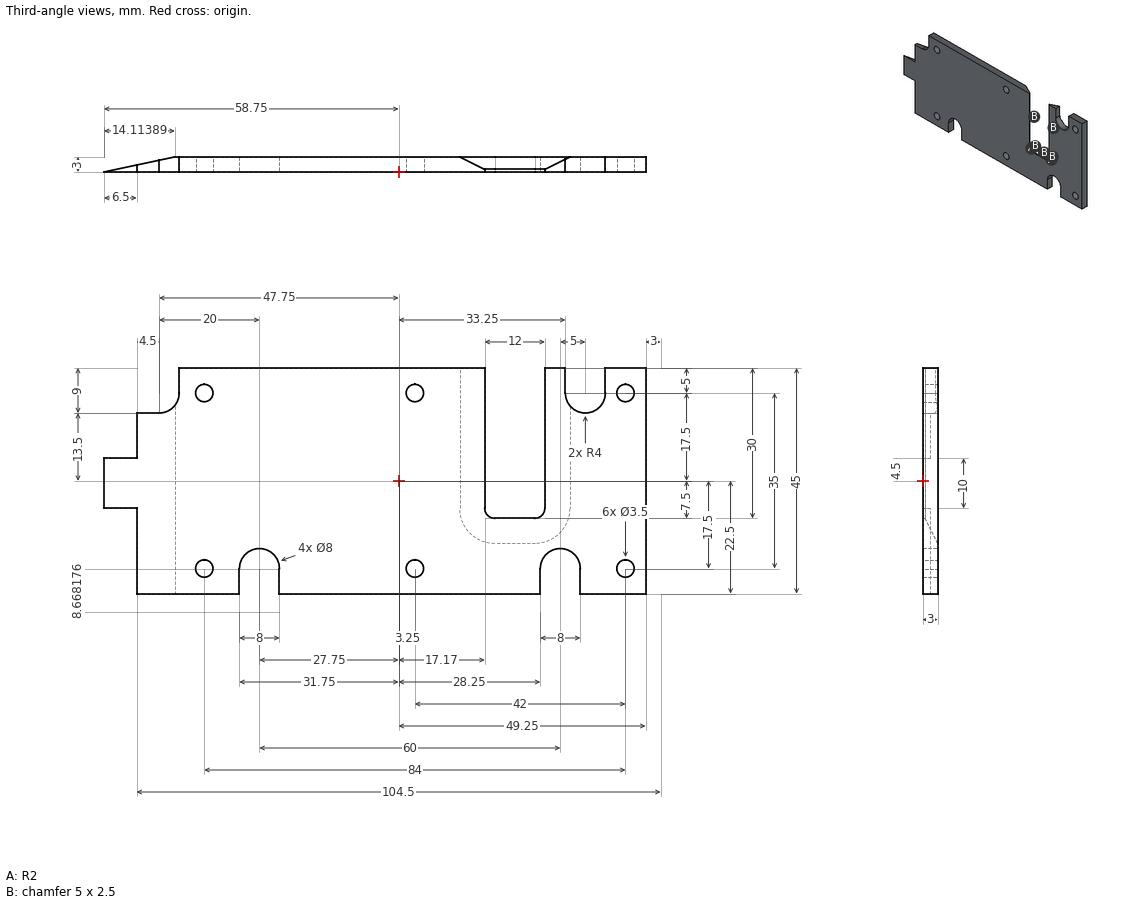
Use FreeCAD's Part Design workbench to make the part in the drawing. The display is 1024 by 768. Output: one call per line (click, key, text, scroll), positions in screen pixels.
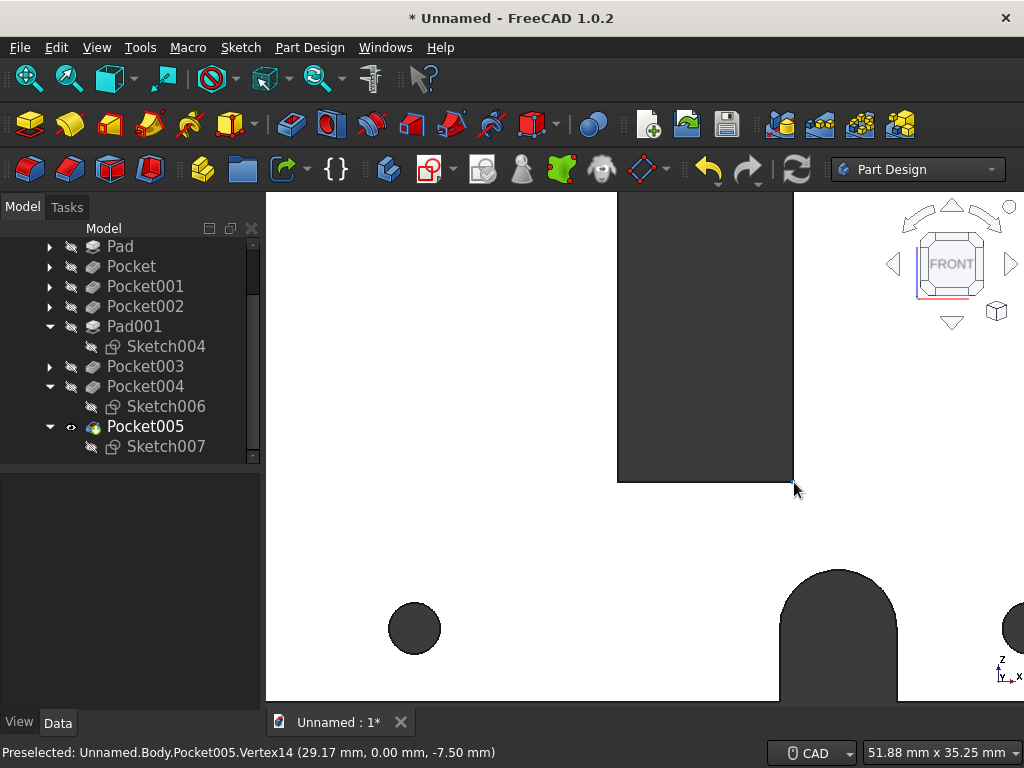
click(30, 80)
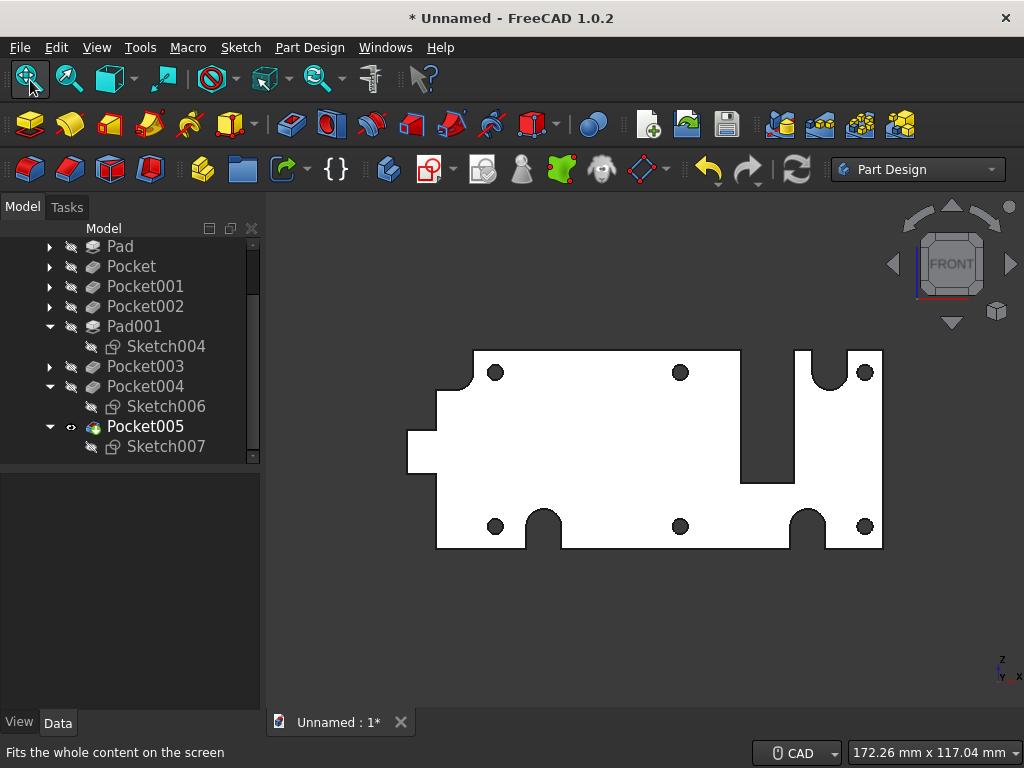
key(3)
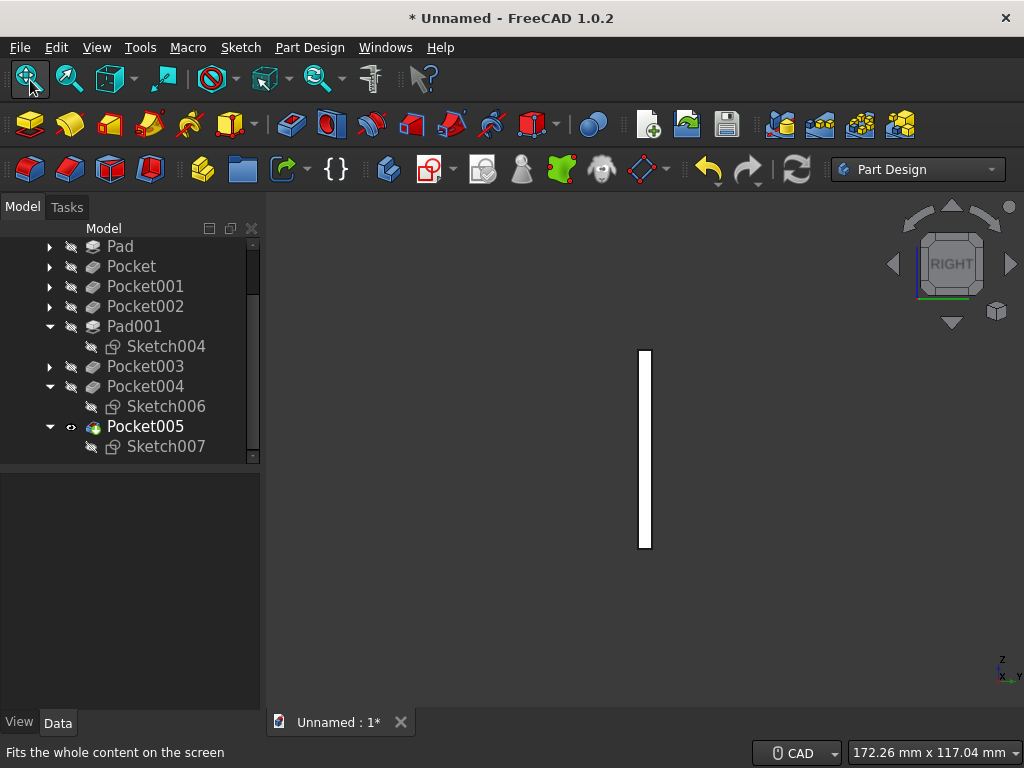
key(v)
key(f)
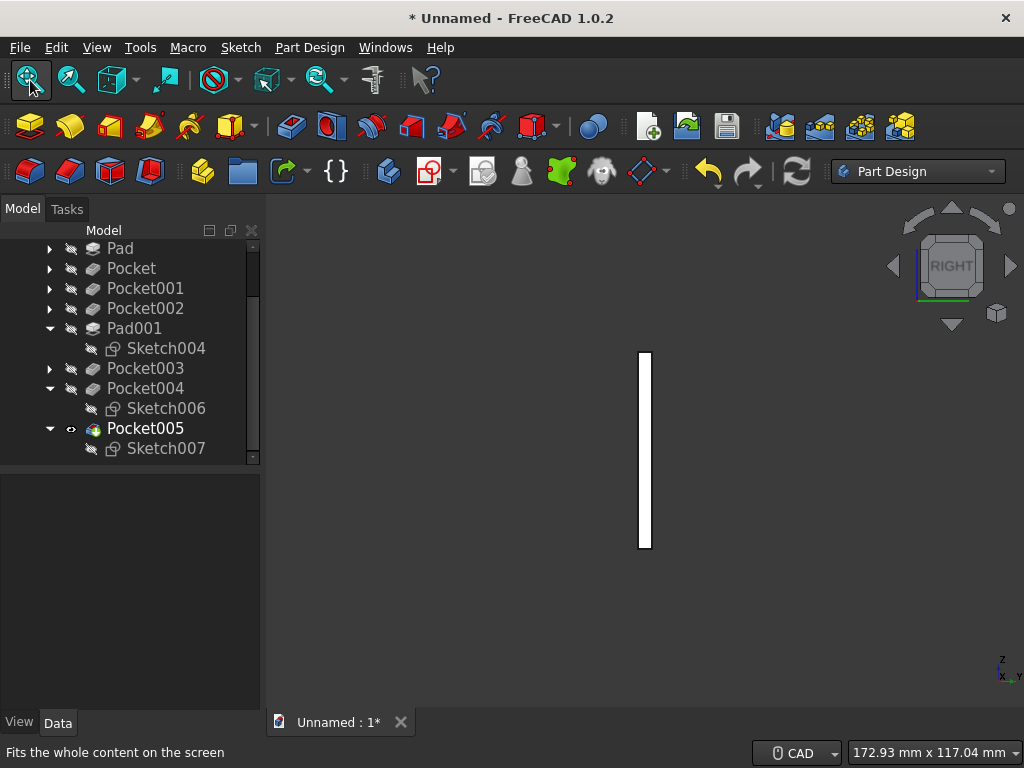
scroll(645, 482, up, 6)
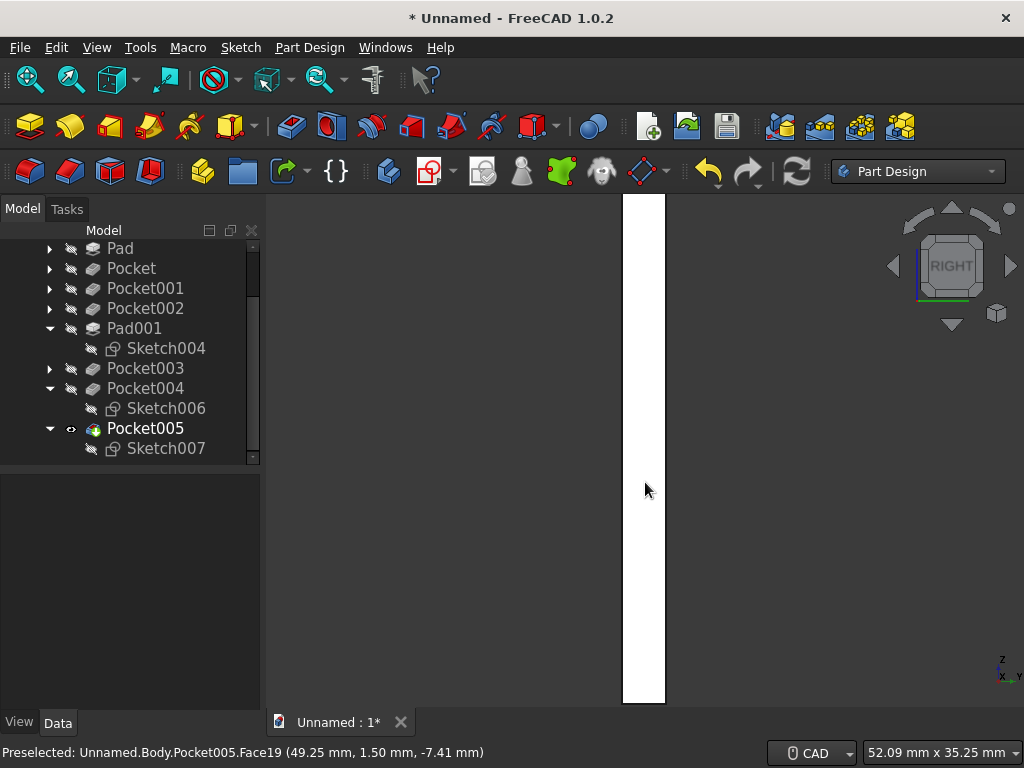
key(v)
key(f)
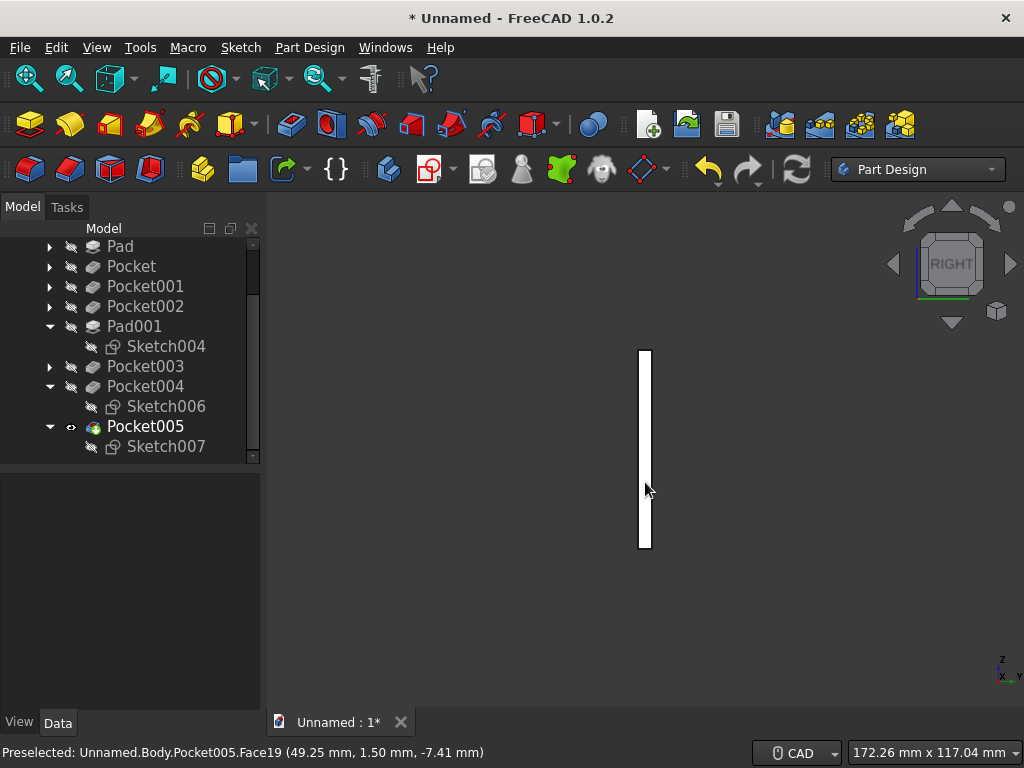
key(5)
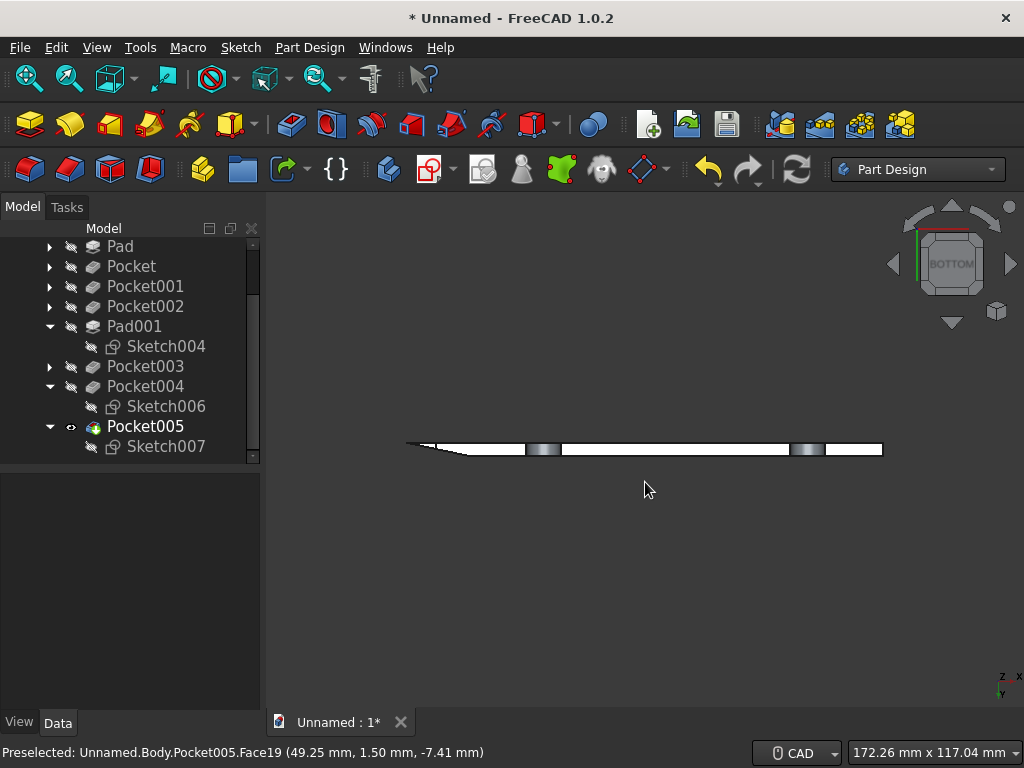
scroll(794, 448, up, 6)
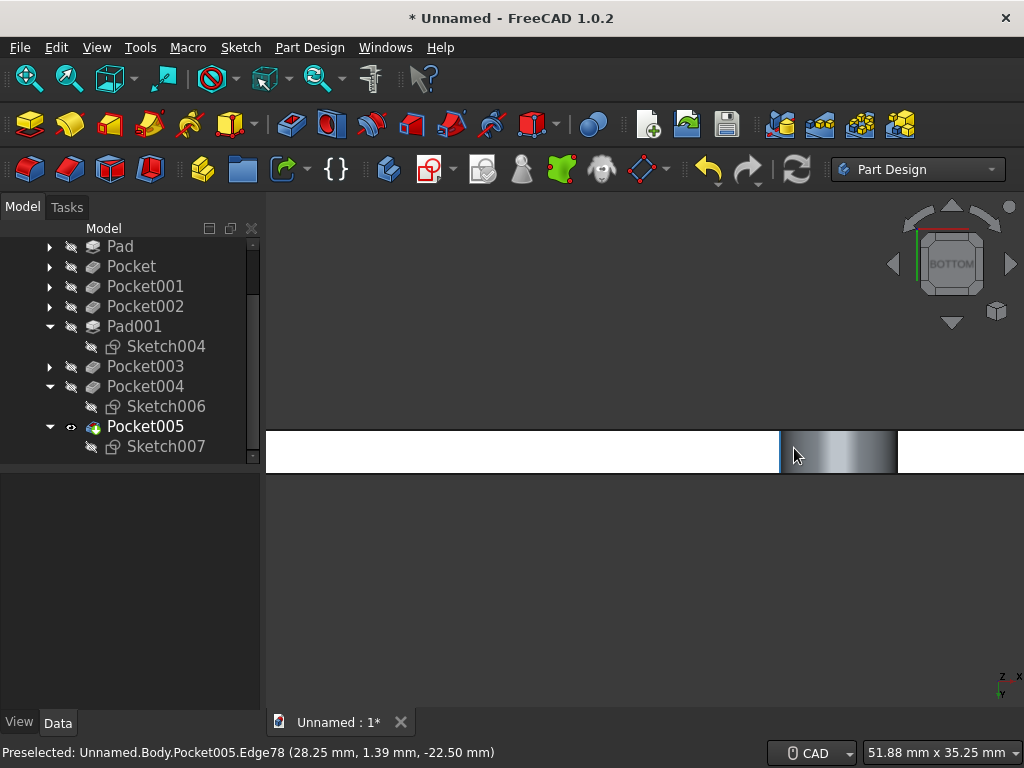
click(30, 80)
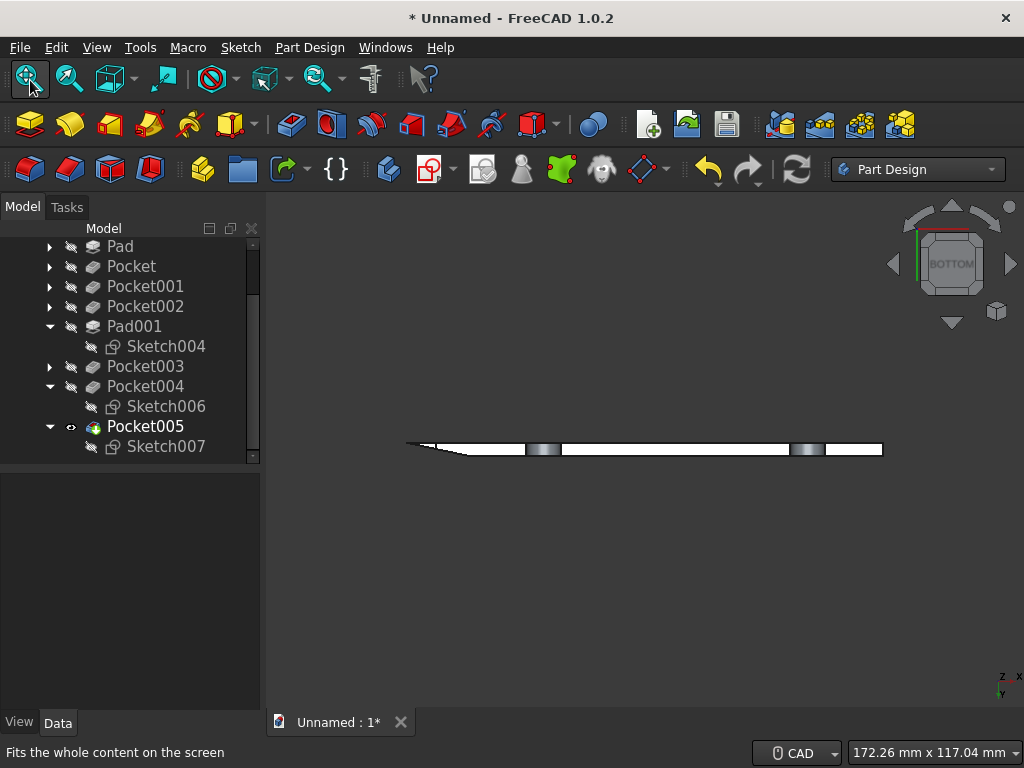
key(4)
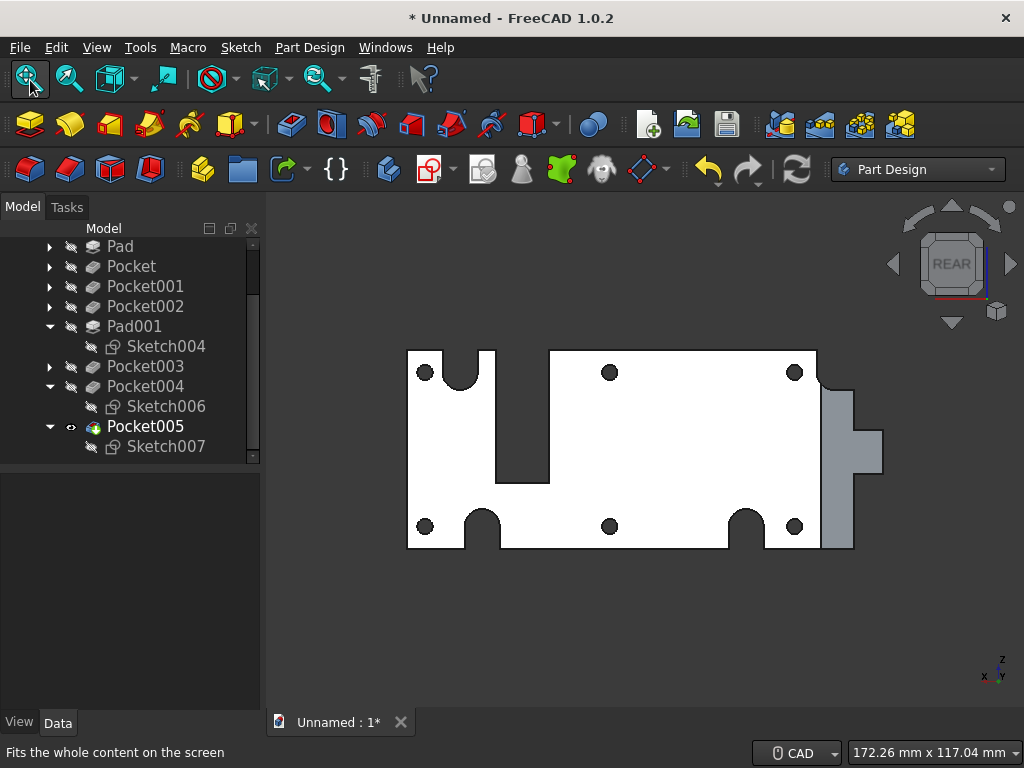
scroll(496, 482, up, 6)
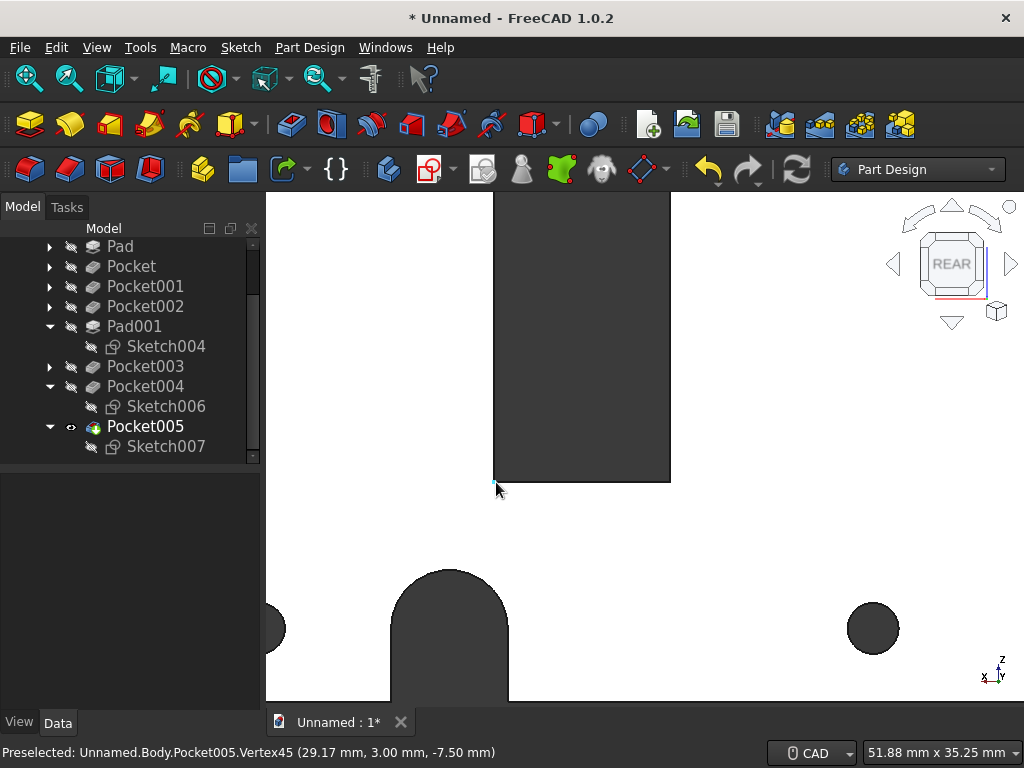
click(30, 80)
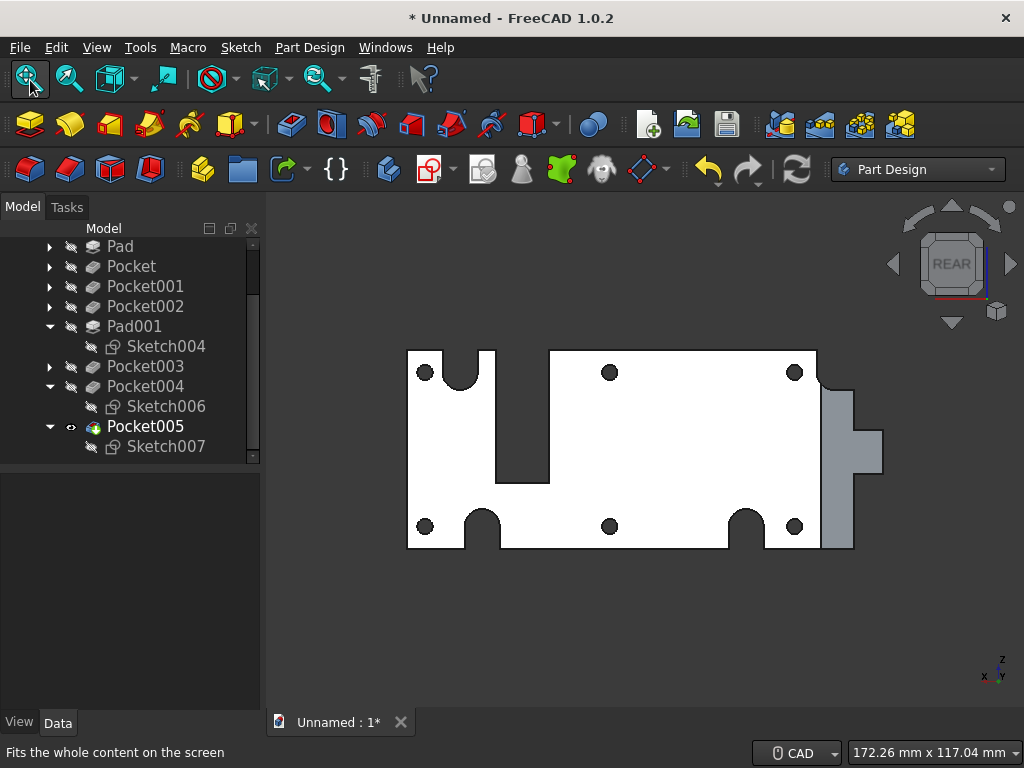
key(6)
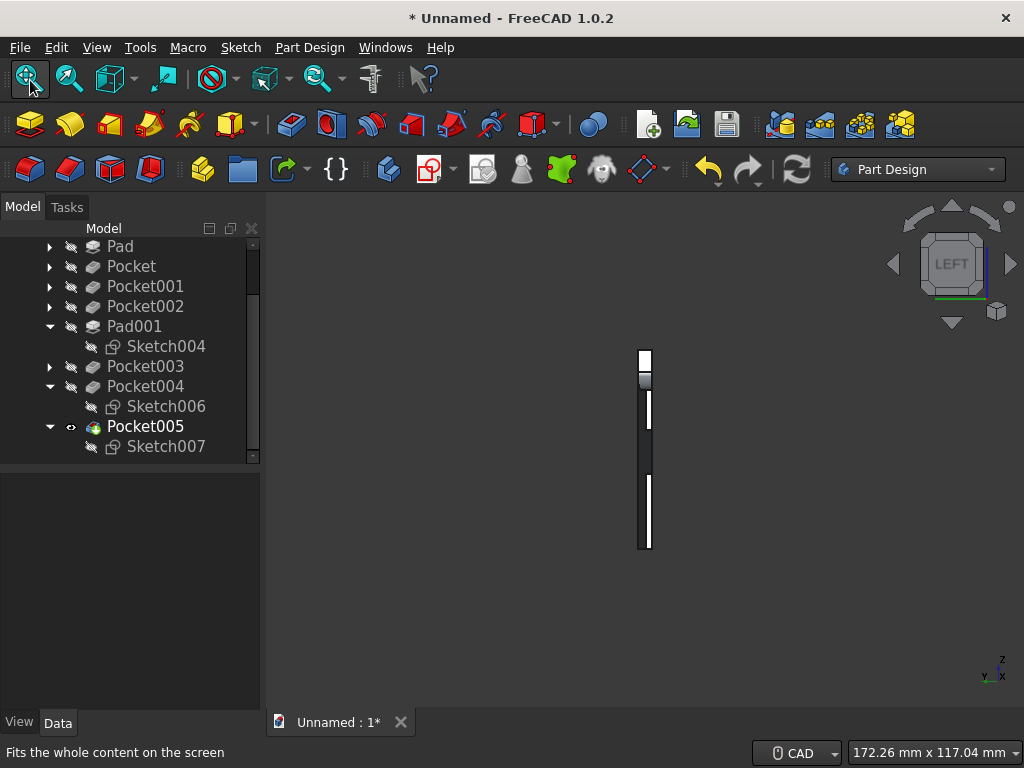
key(v)
key(f)